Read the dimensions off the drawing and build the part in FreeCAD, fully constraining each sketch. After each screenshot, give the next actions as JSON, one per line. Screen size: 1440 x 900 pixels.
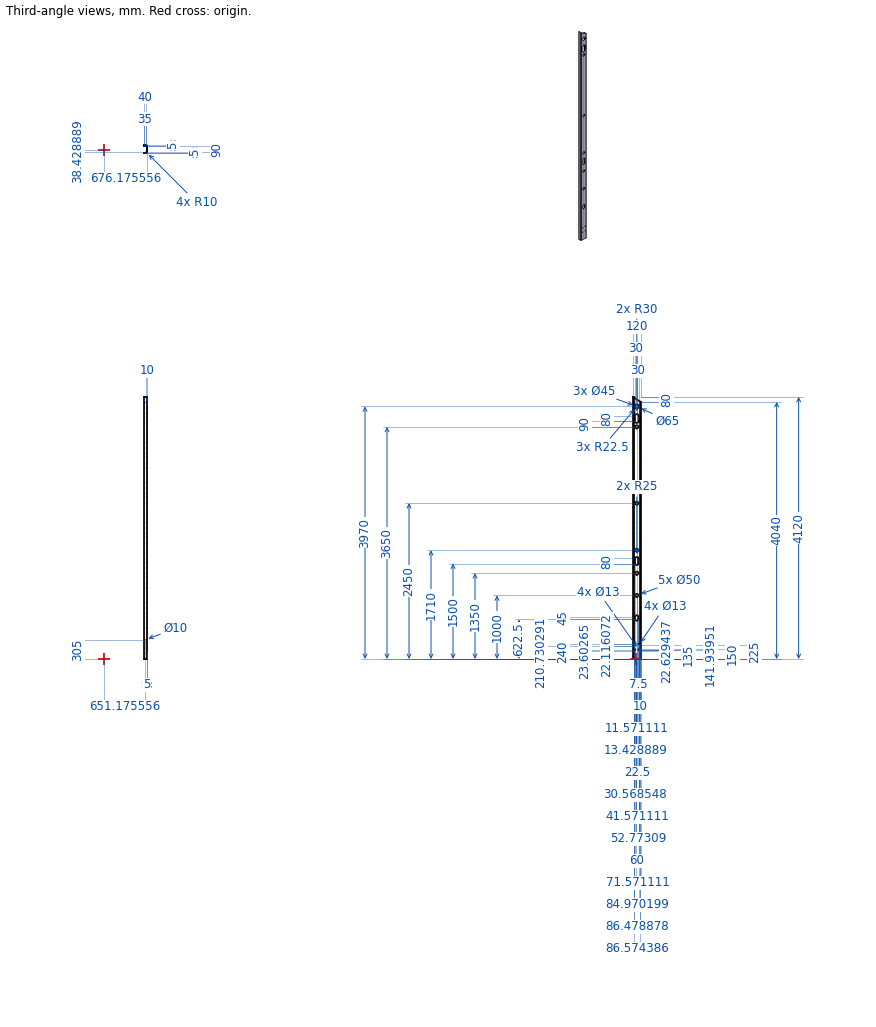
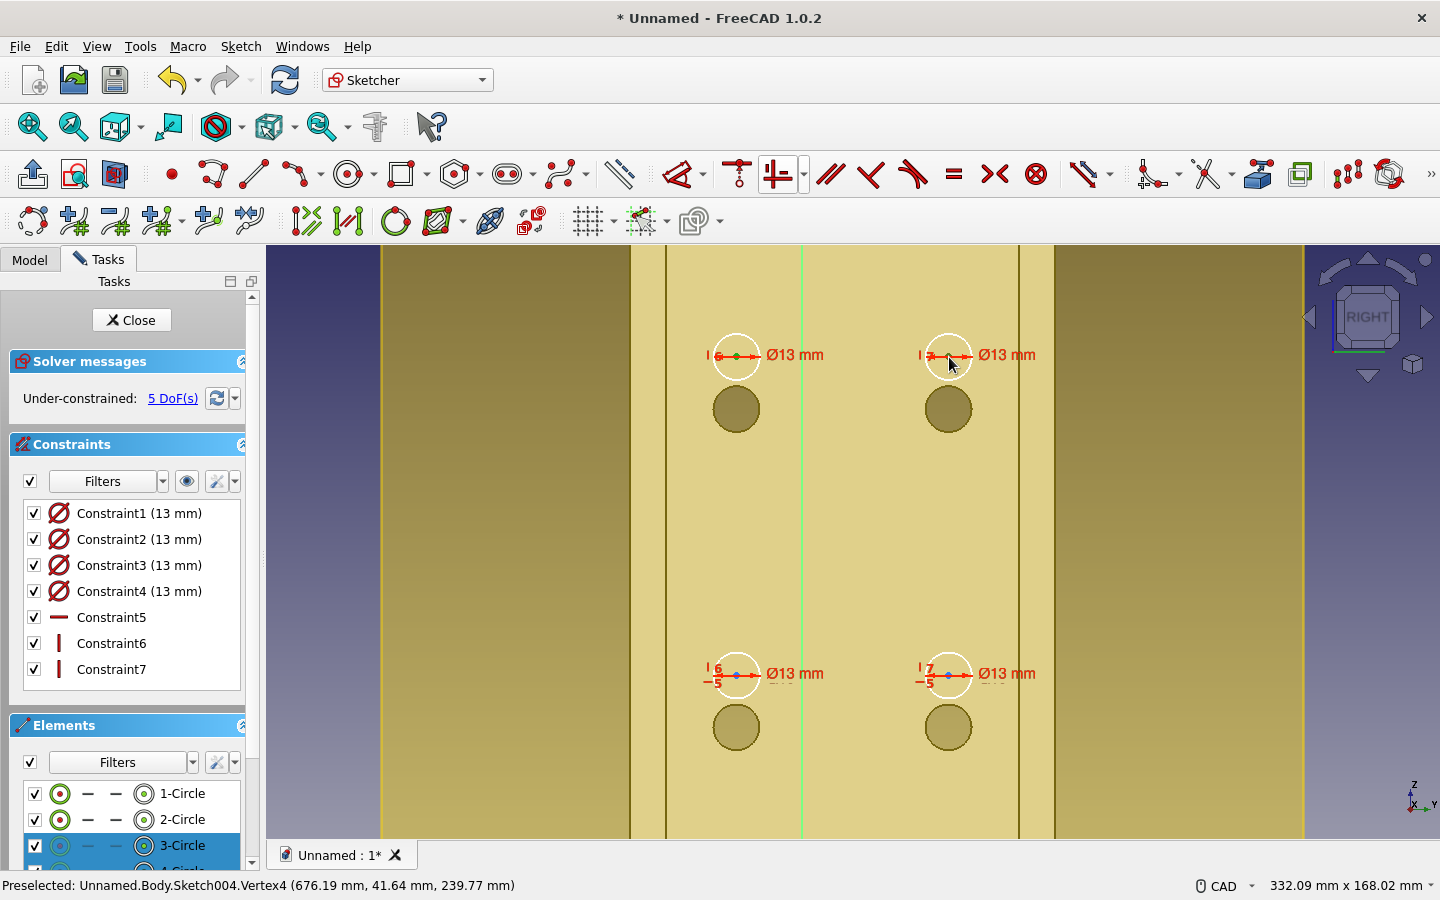
{"action": "key", "text": "h"}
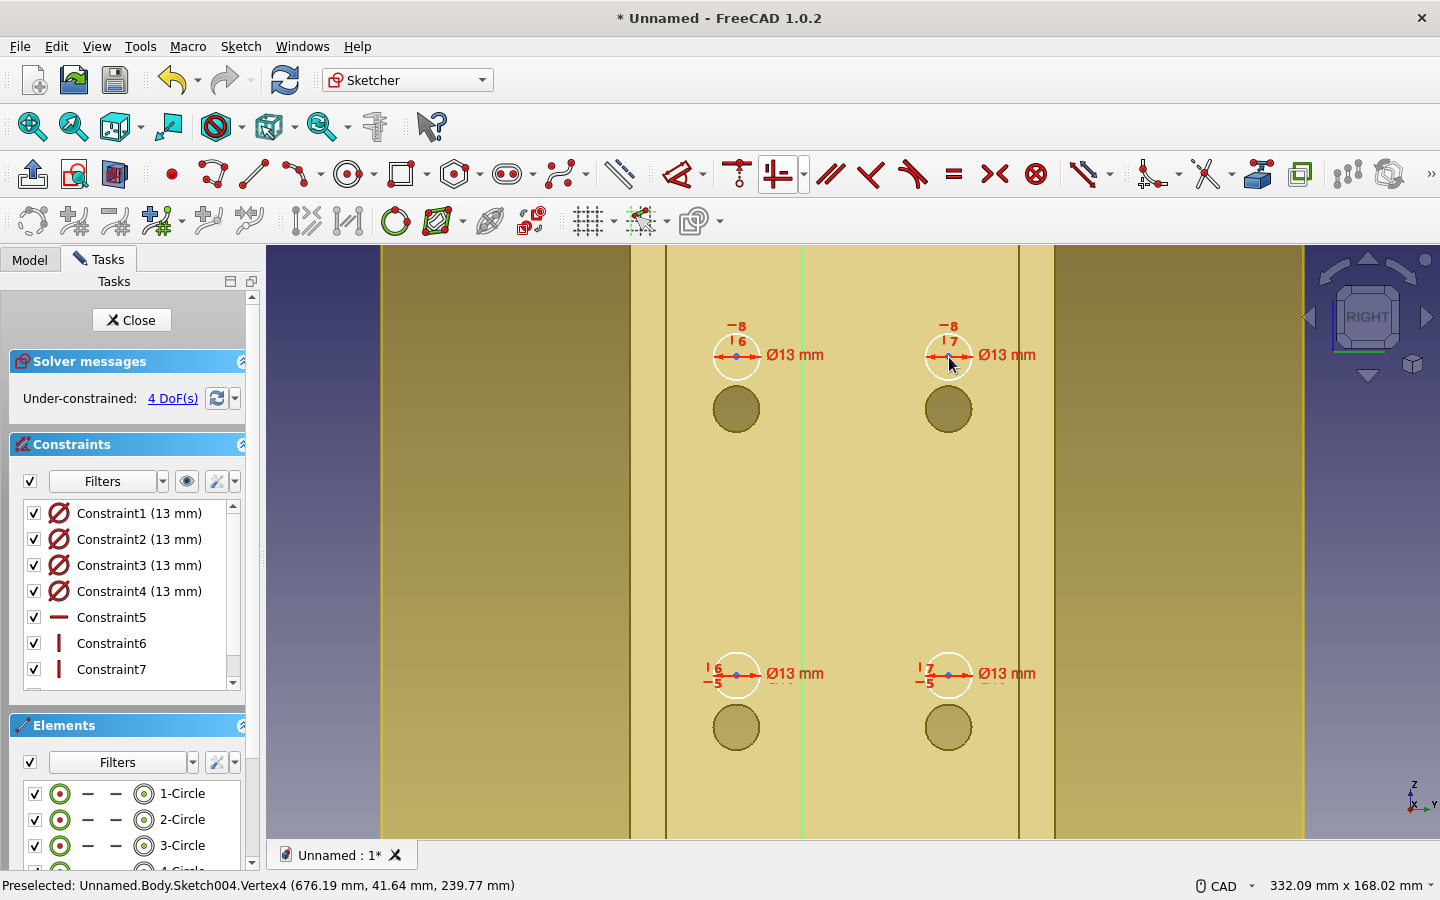
{"action": "key", "text": "d"}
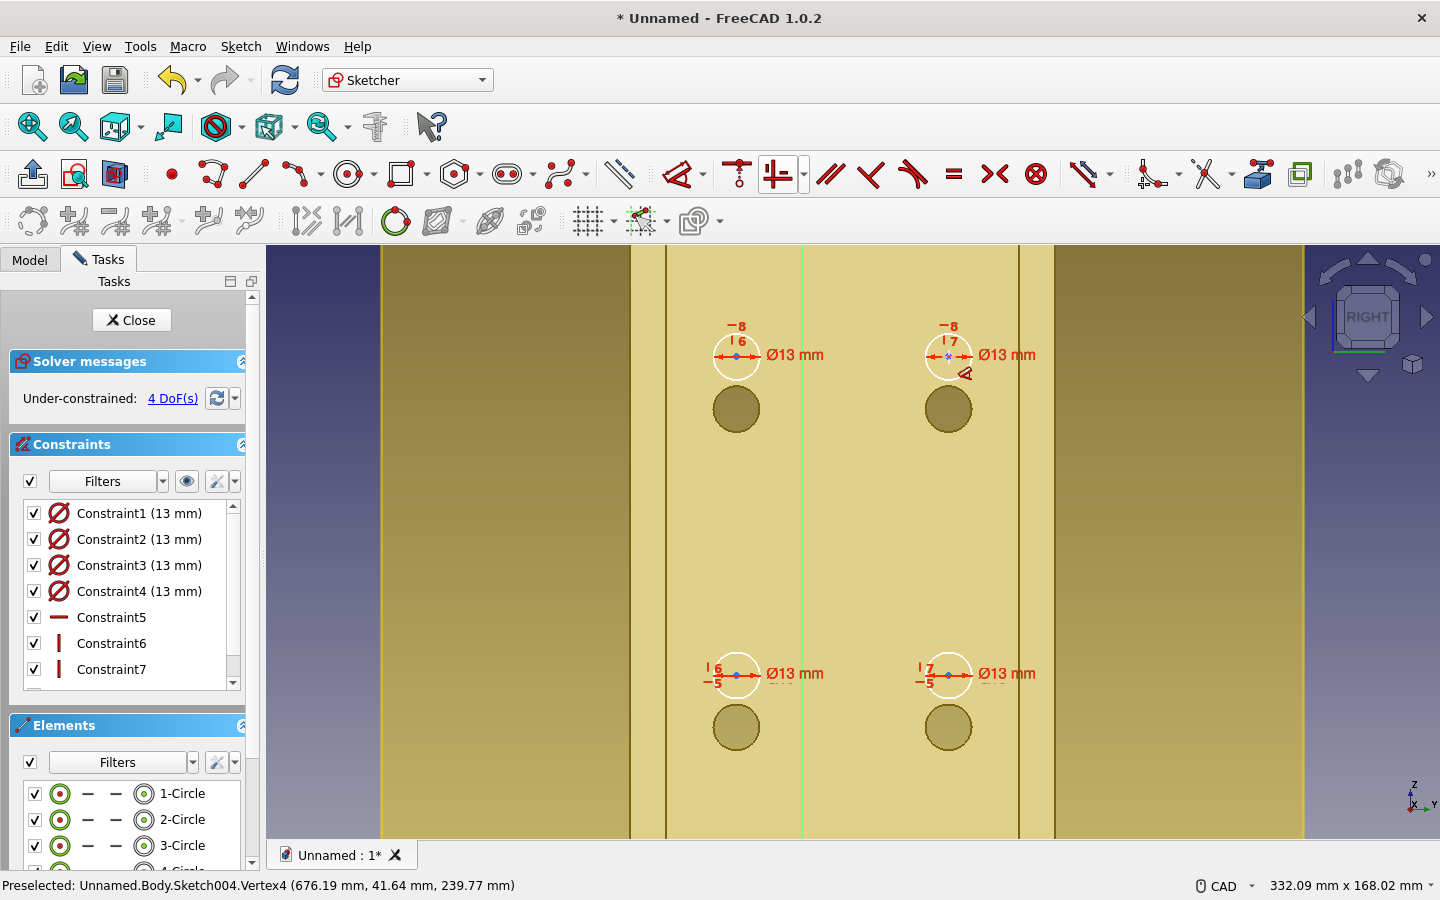
{"action": "left_click", "coordinate": [949, 676]}
{"action": "left_click", "coordinate": [983, 743]}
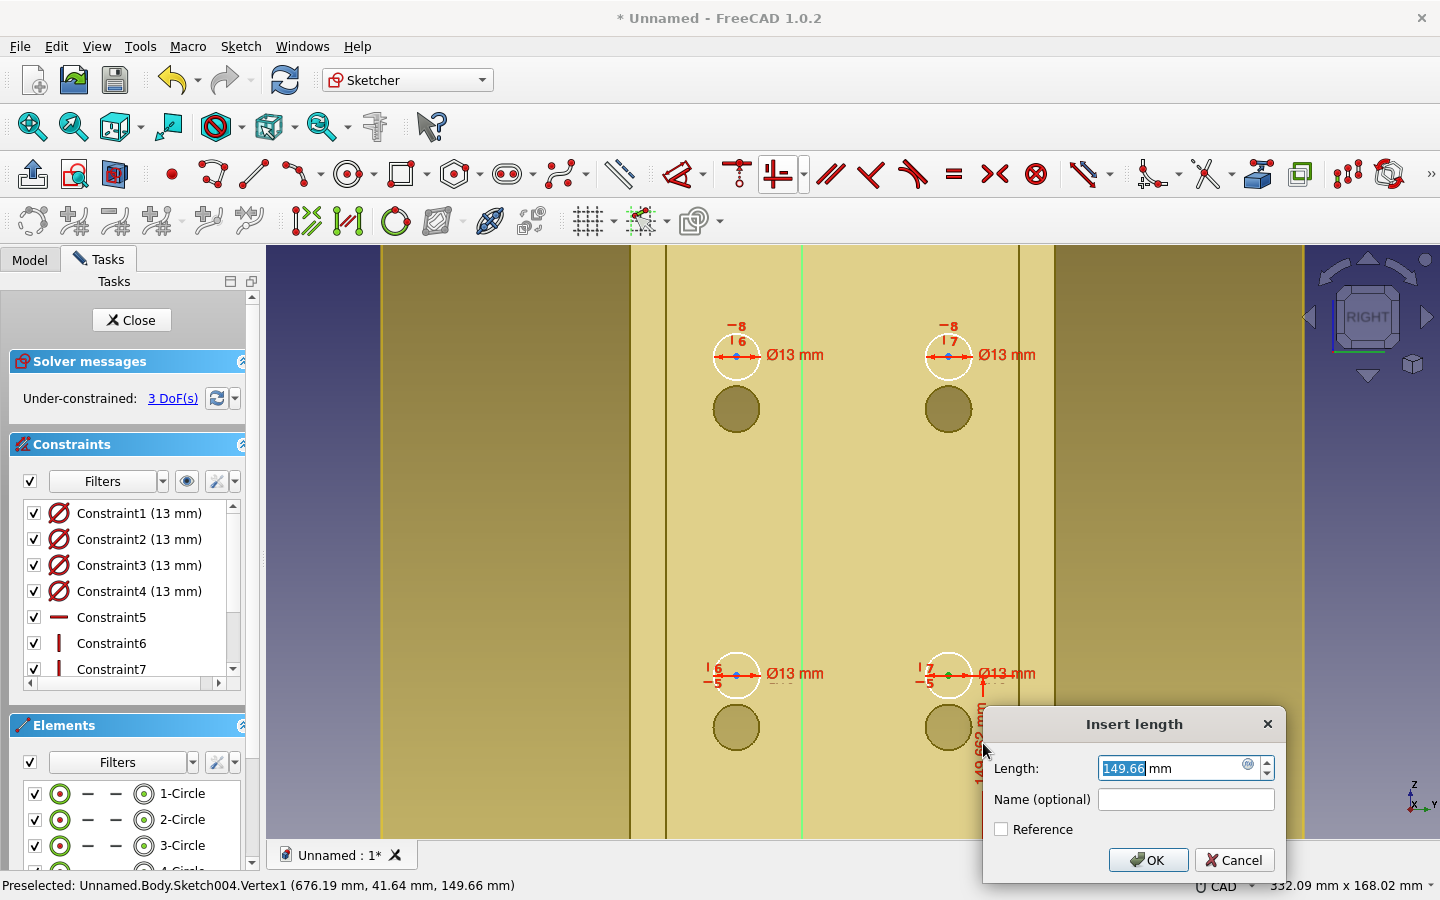
{"action": "type", "text": "150"}
{"action": "key", "text": "Return"}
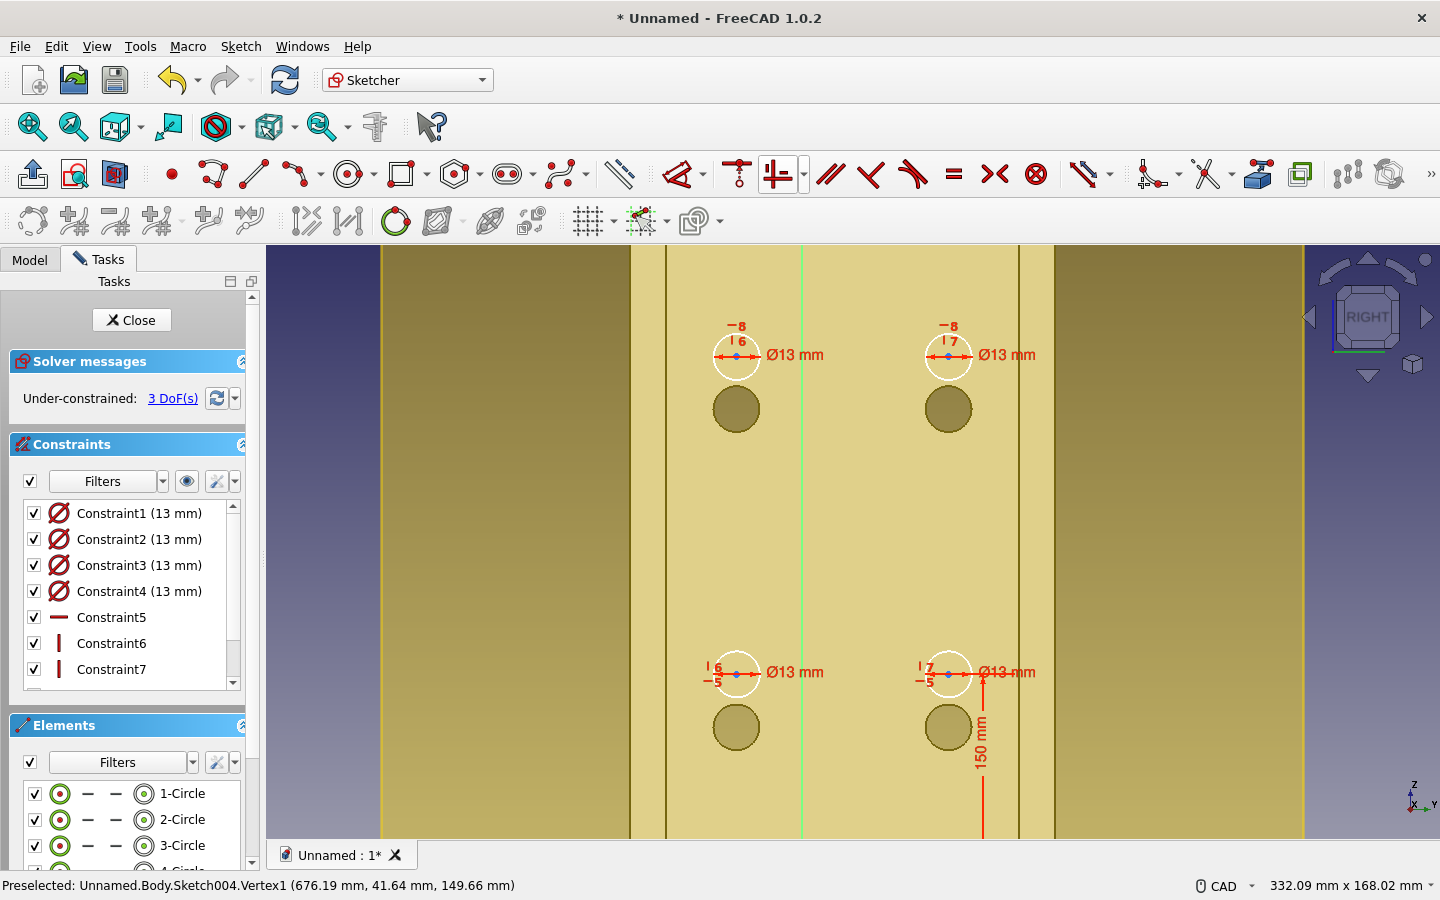
{"action": "left_click", "coordinate": [737, 357]}
{"action": "left_click", "coordinate": [703, 584]}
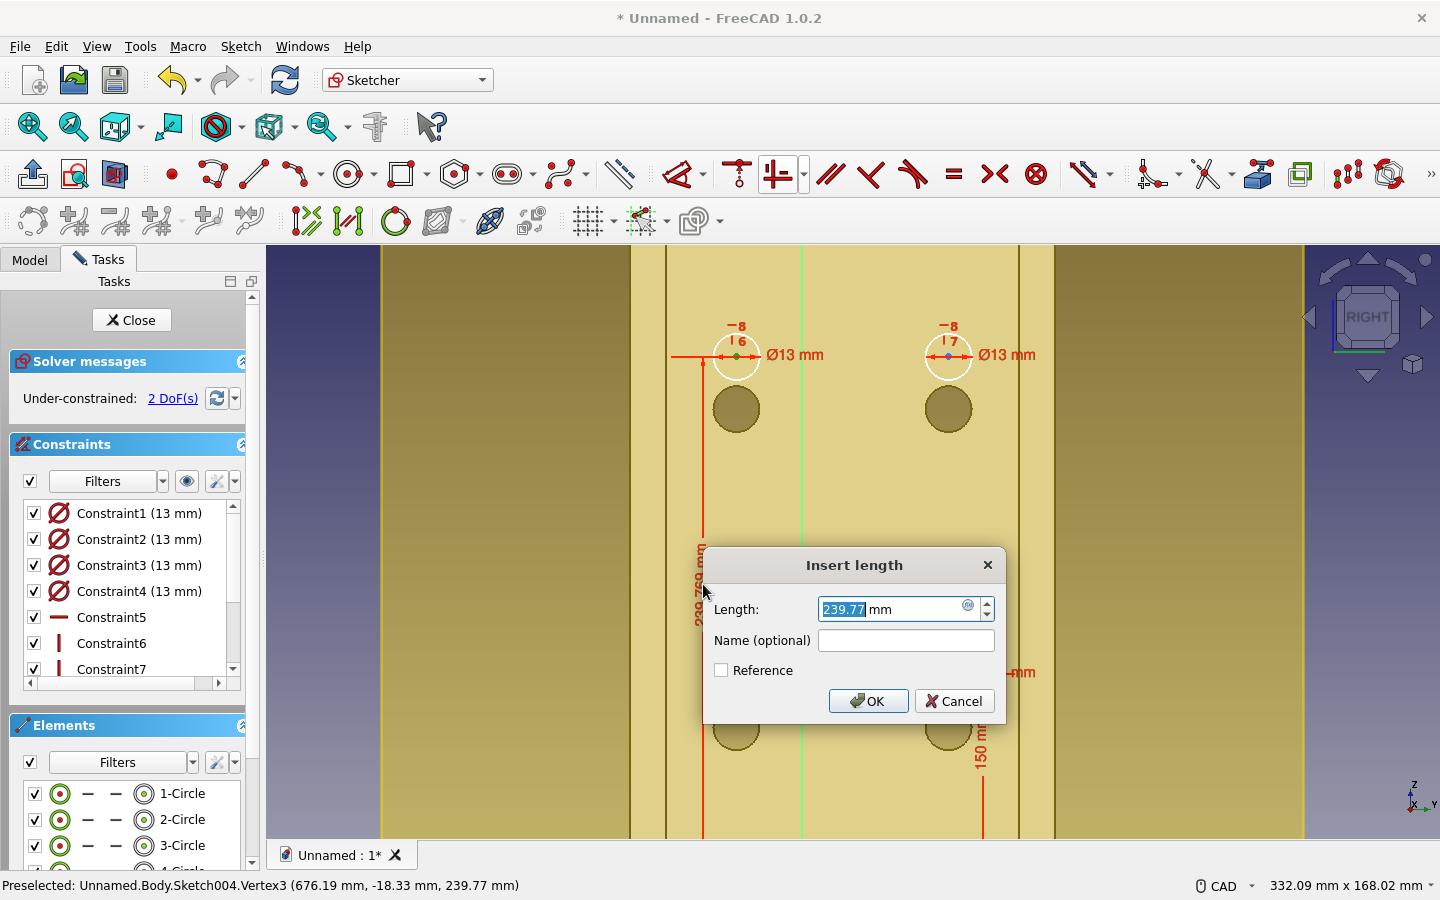
{"action": "type", "text": "240"}
{"action": "key", "text": "Return"}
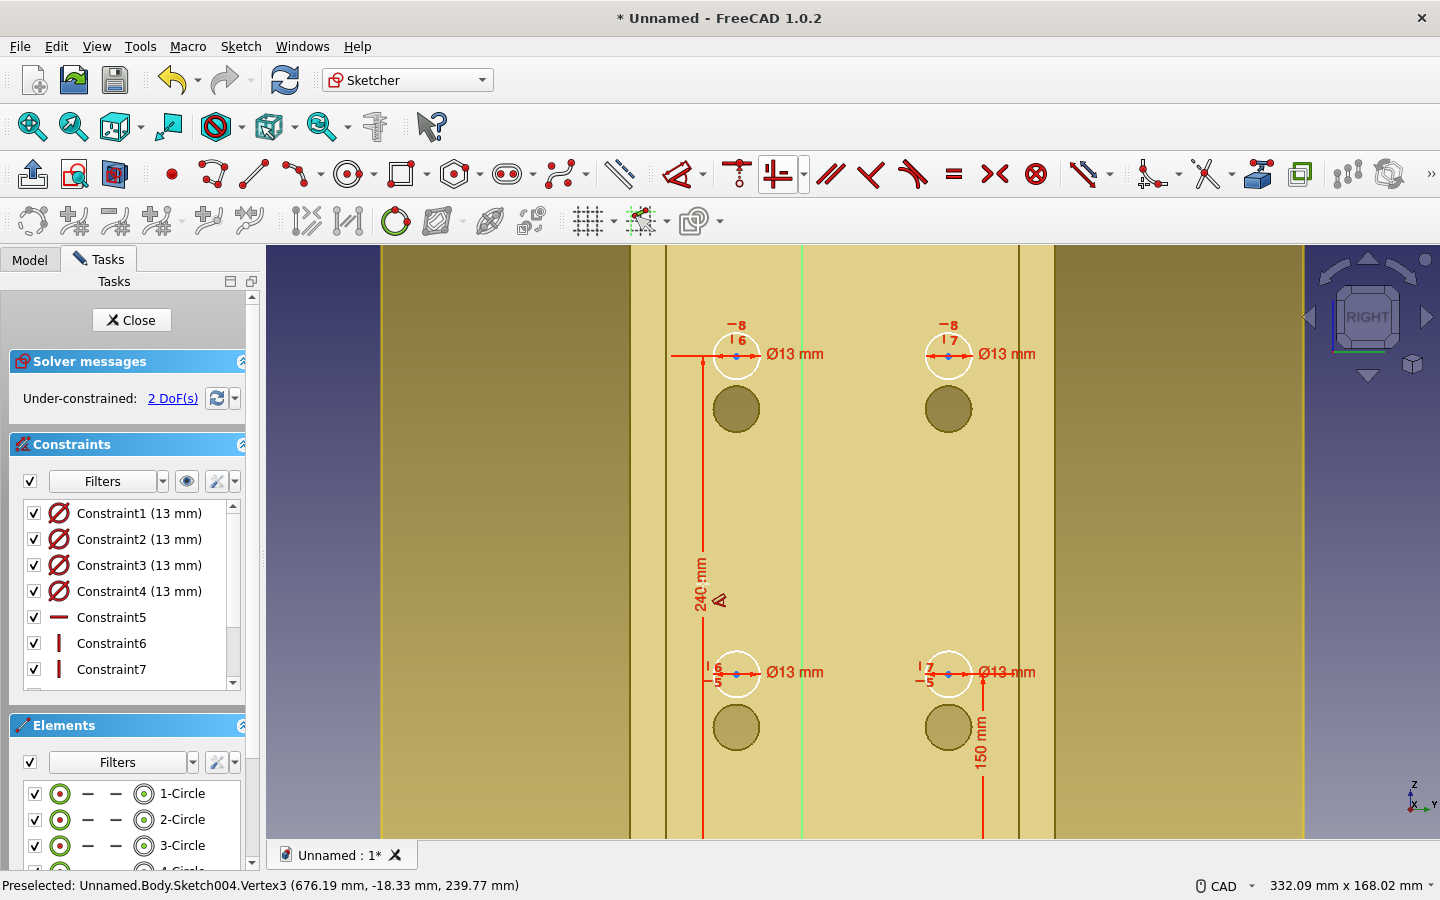
{"action": "left_click", "coordinate": [949, 674]}